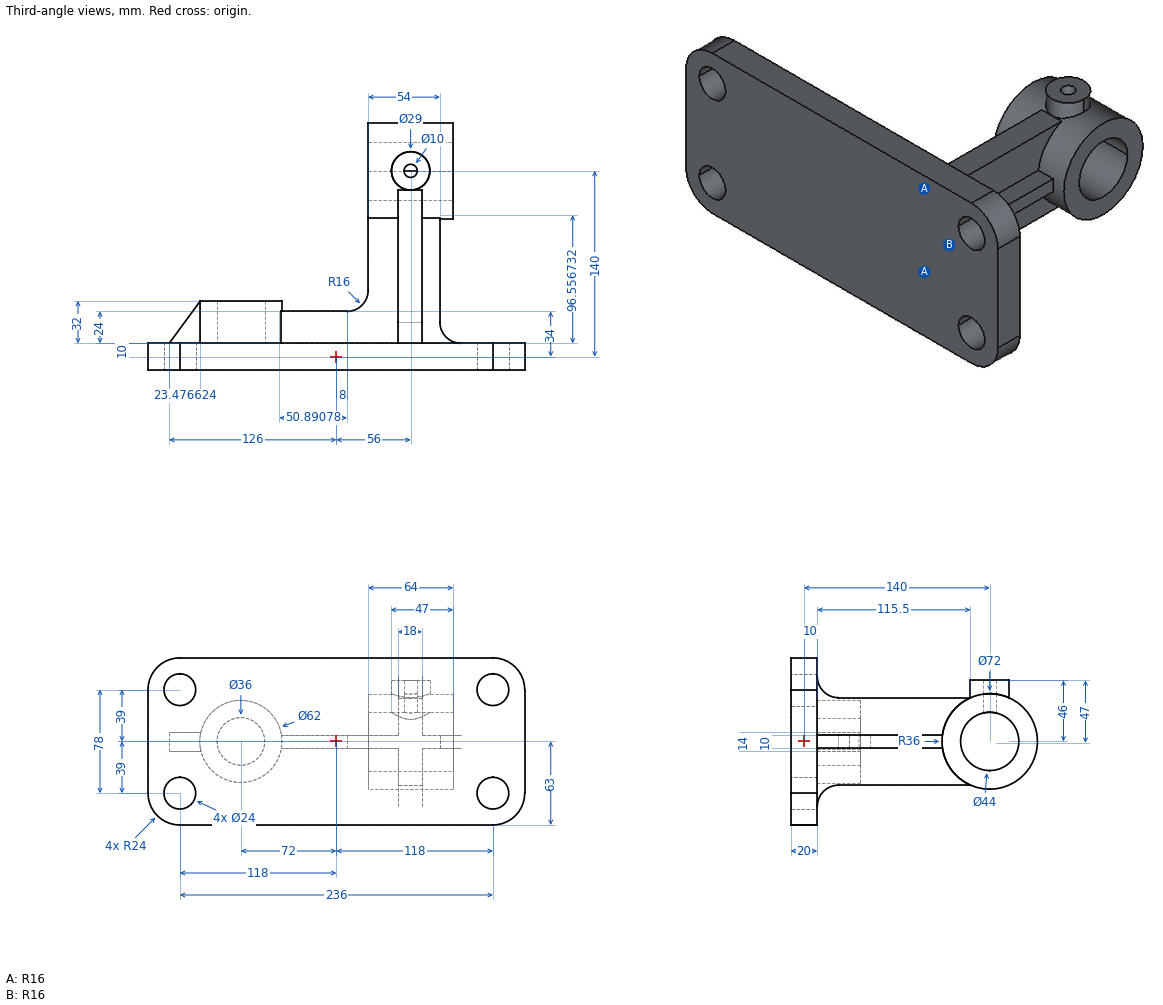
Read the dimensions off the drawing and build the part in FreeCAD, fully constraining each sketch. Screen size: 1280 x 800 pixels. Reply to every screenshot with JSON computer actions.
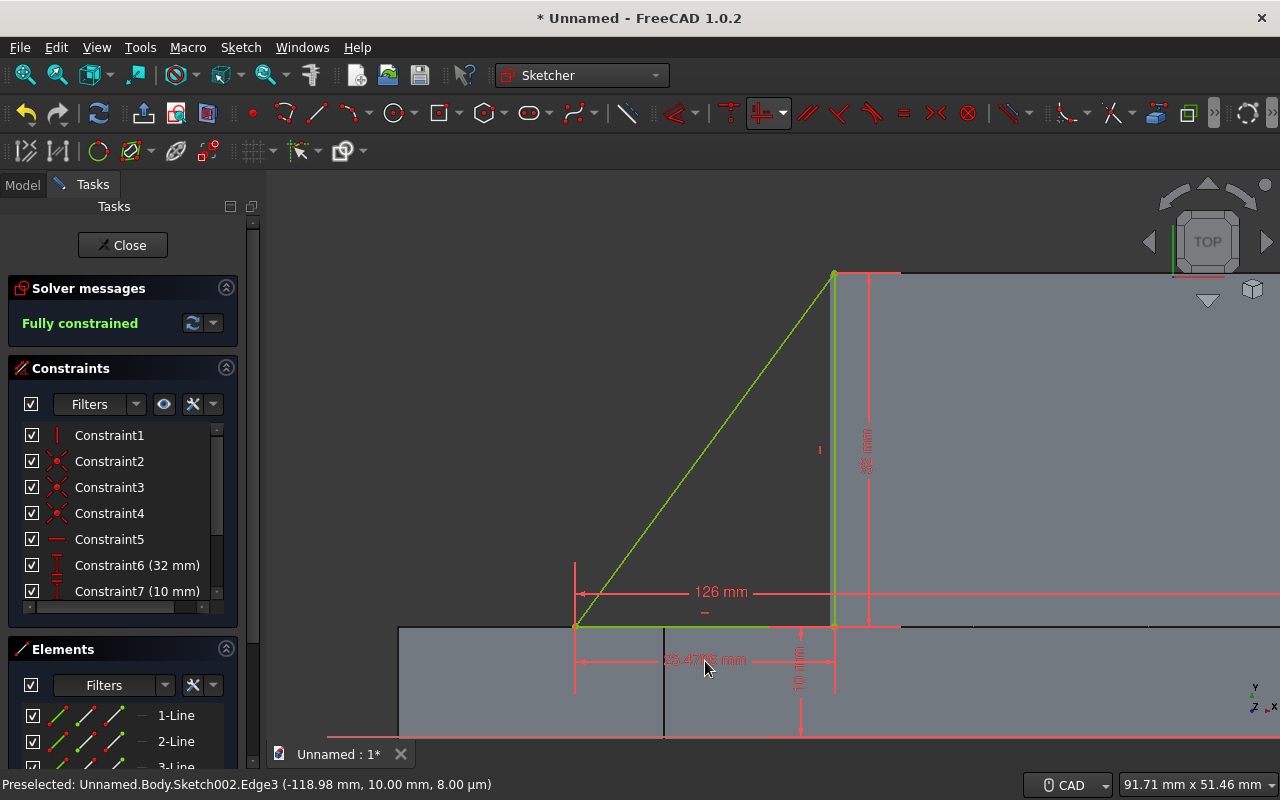
{"action": "left_click", "coordinate": [123, 245]}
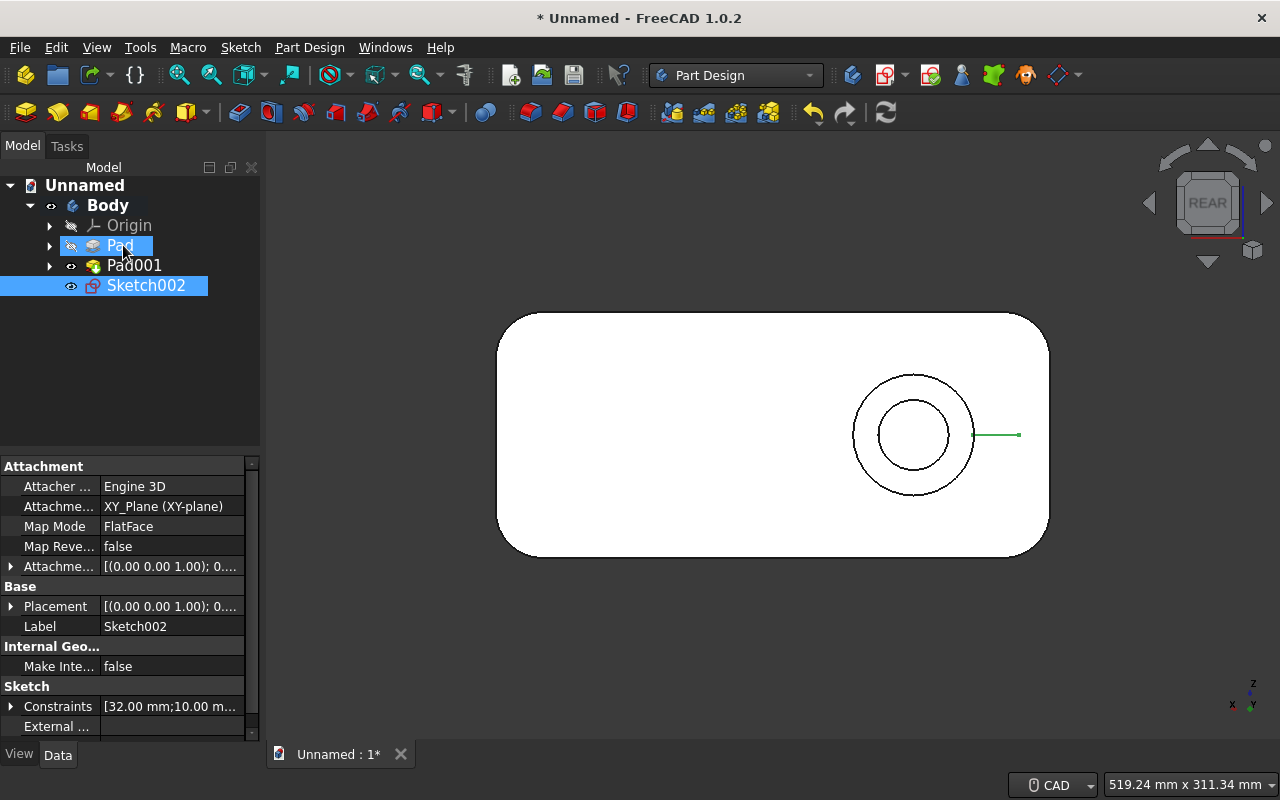
{"action": "left_click", "coordinate": [26, 112]}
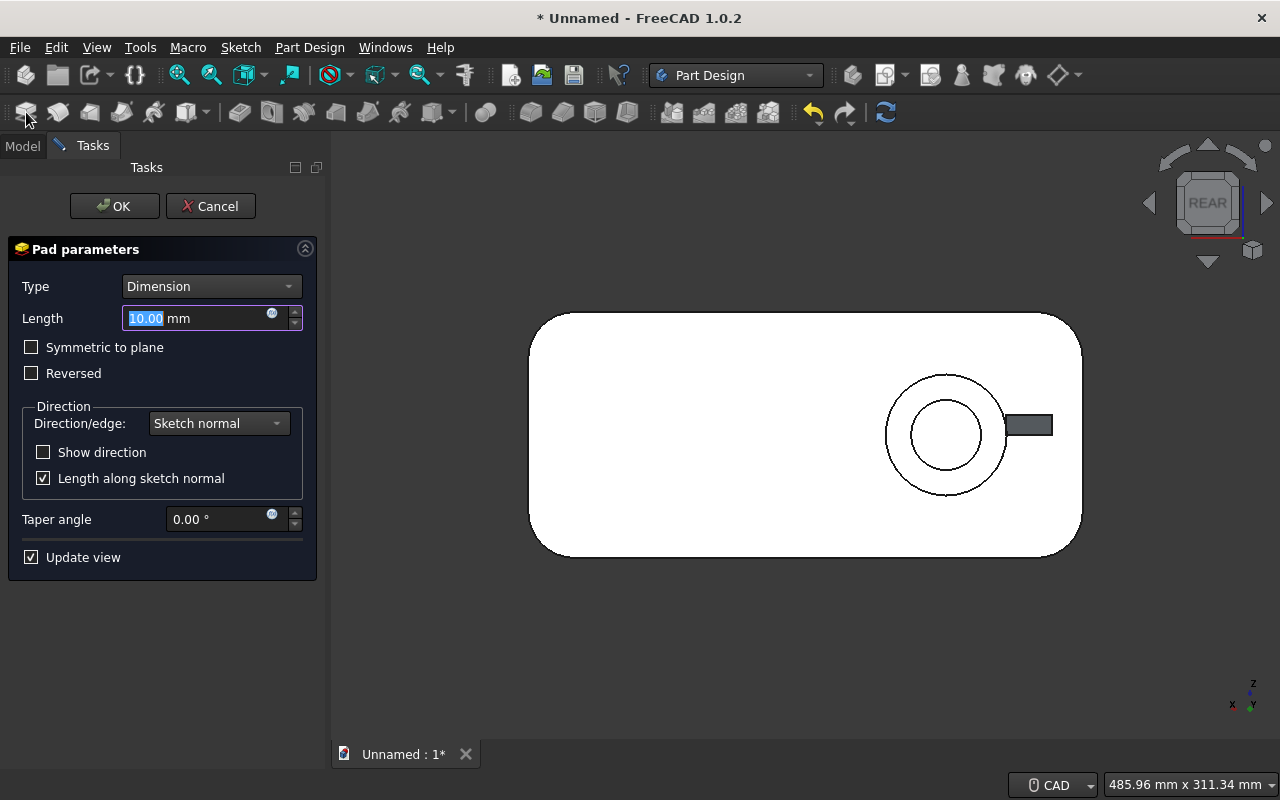
{"action": "type", "text": "14"}
{"action": "key", "text": "Tab"}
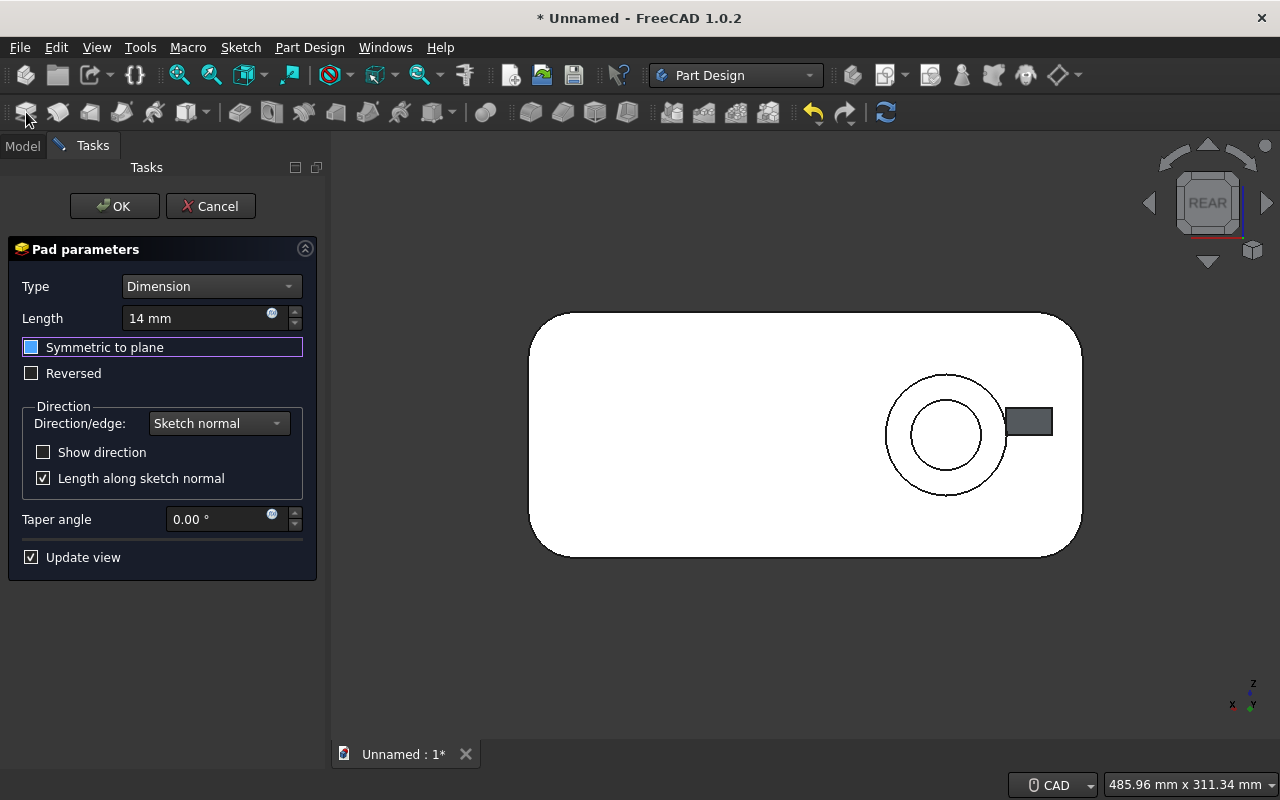
{"action": "left_click", "coordinate": [30, 347]}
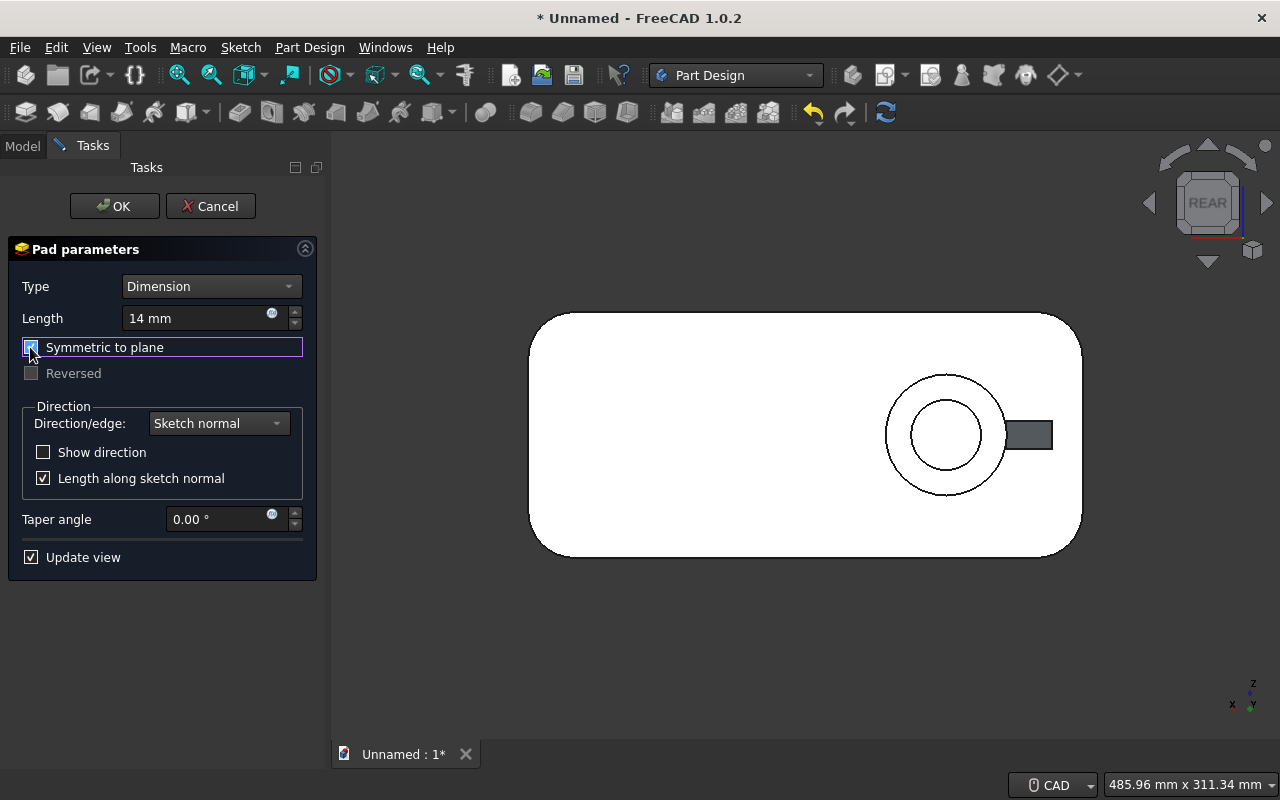
{"action": "left_click", "coordinate": [115, 206]}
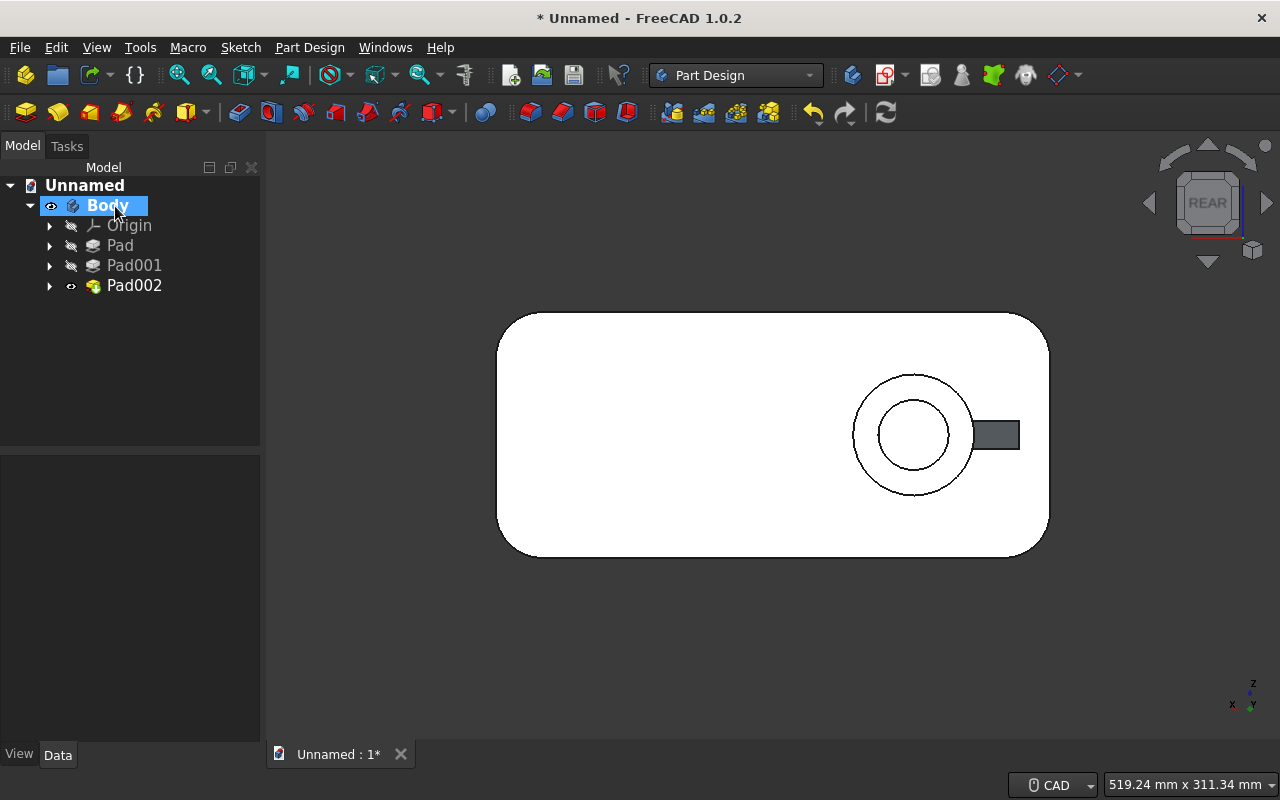
{"action": "left_click", "coordinate": [854, 76]}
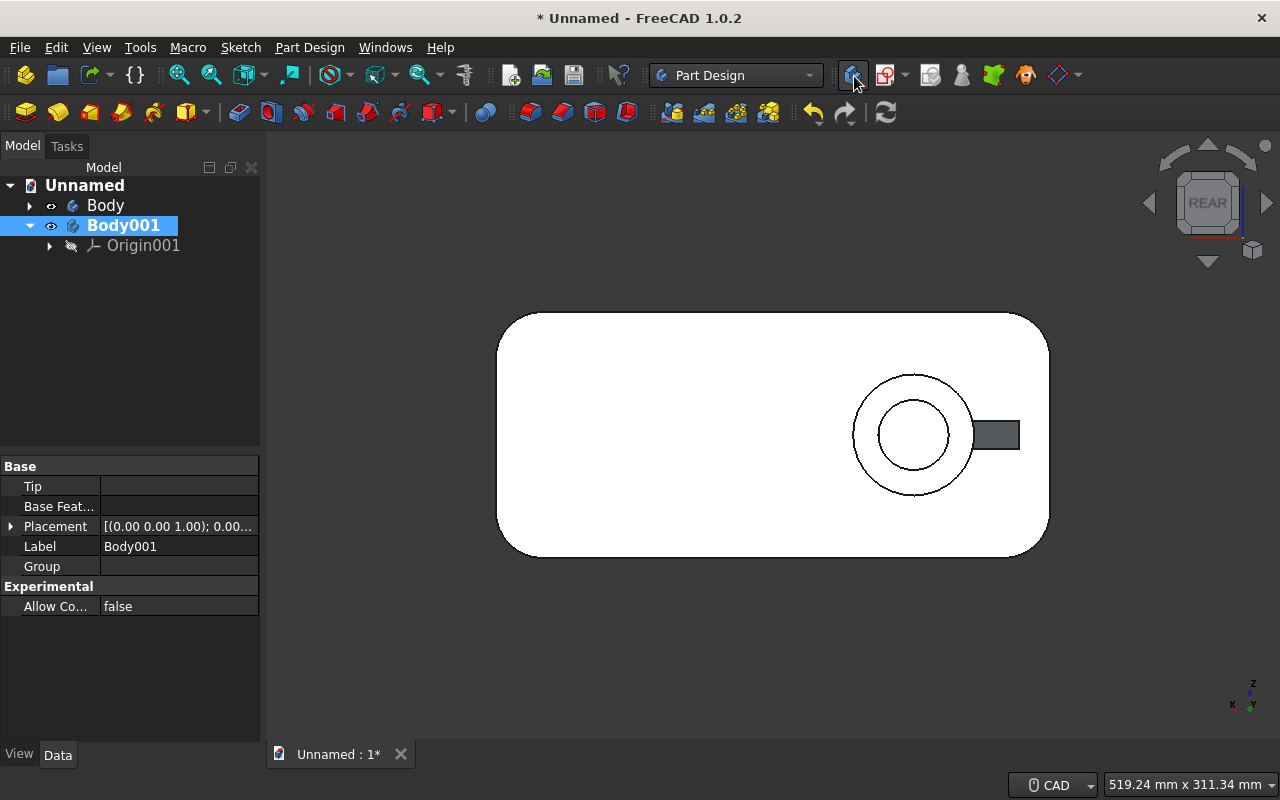
{"action": "left_click", "coordinate": [50, 246]}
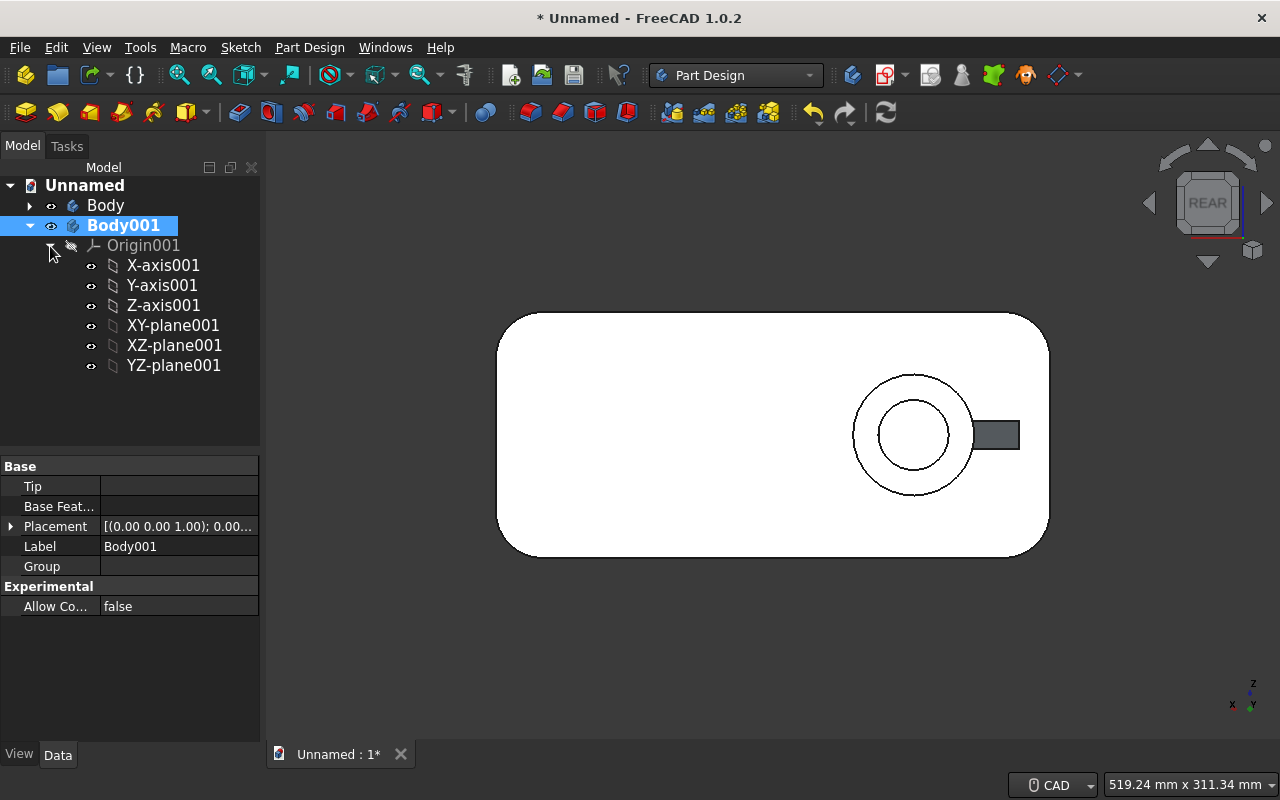
{"action": "left_click", "coordinate": [136, 366]}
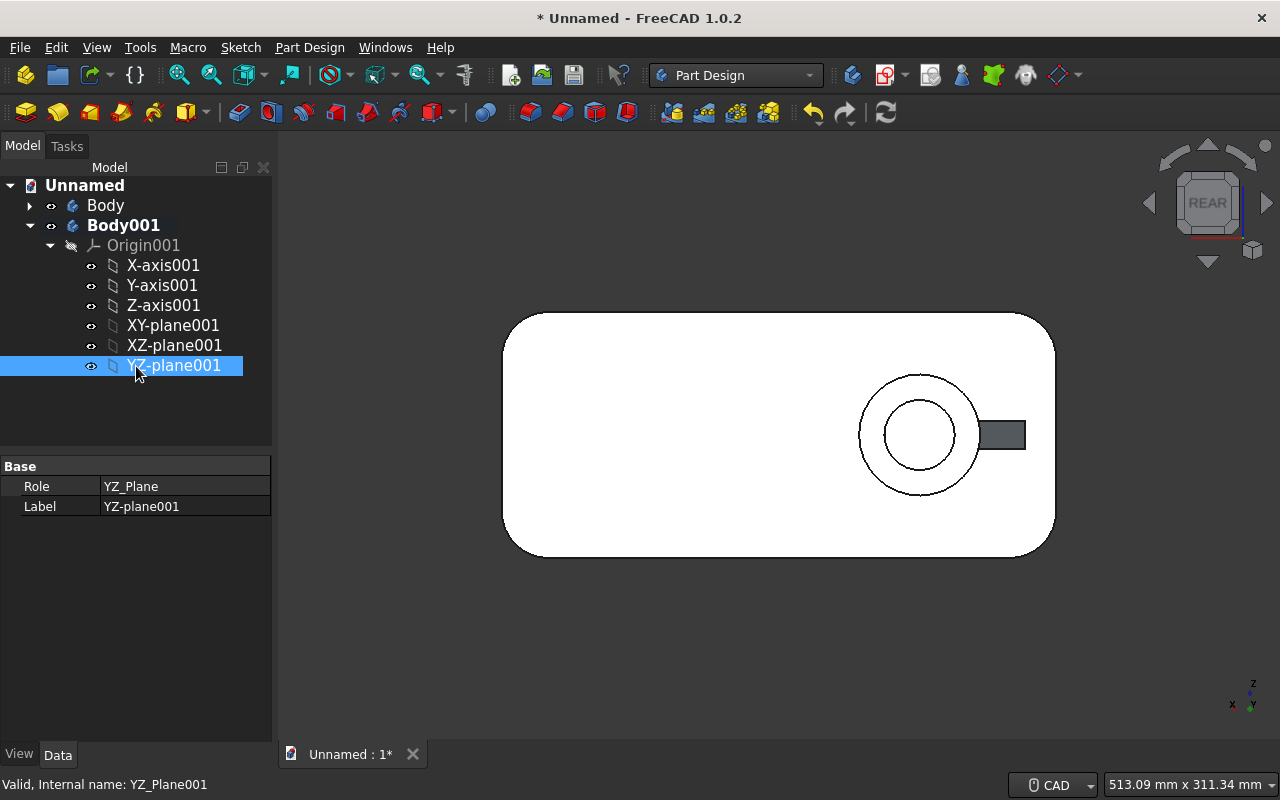
{"action": "left_click", "coordinate": [1058, 76]}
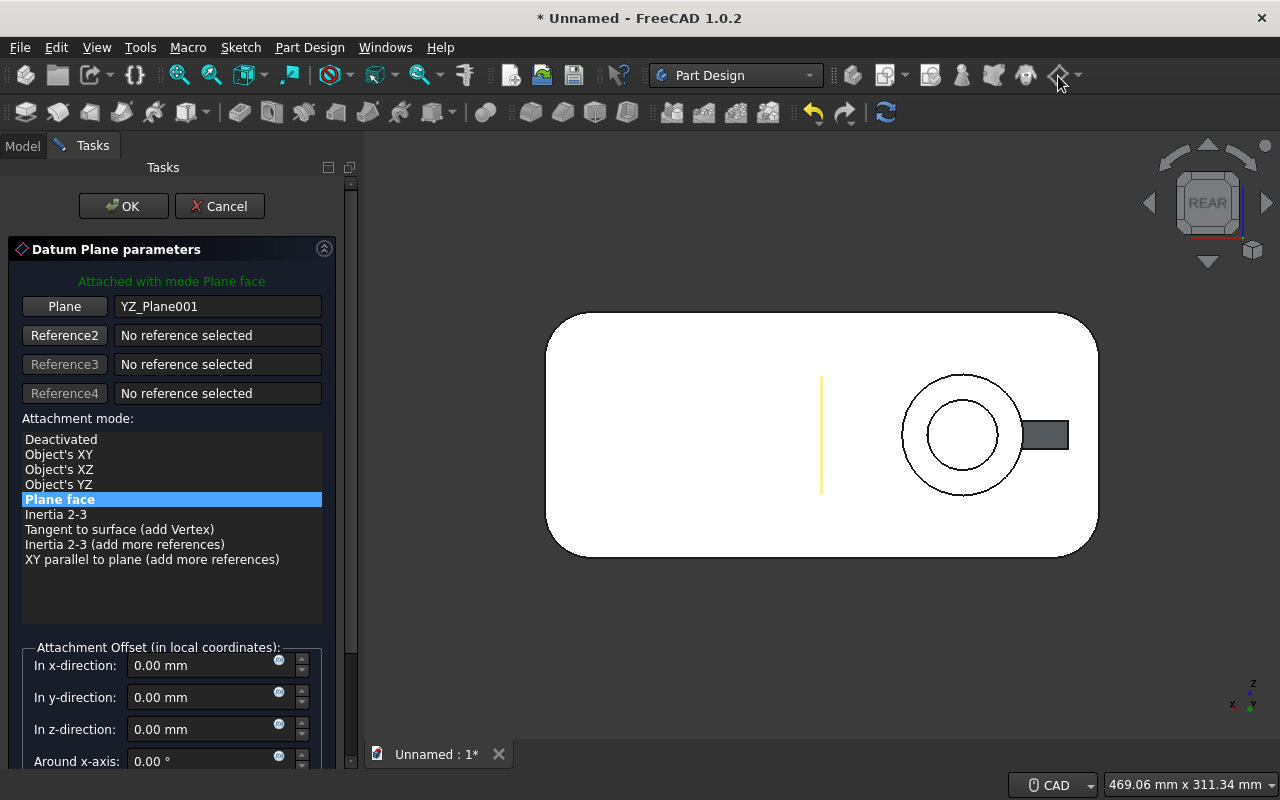
{"action": "triple_click", "coordinate": [210, 729]}